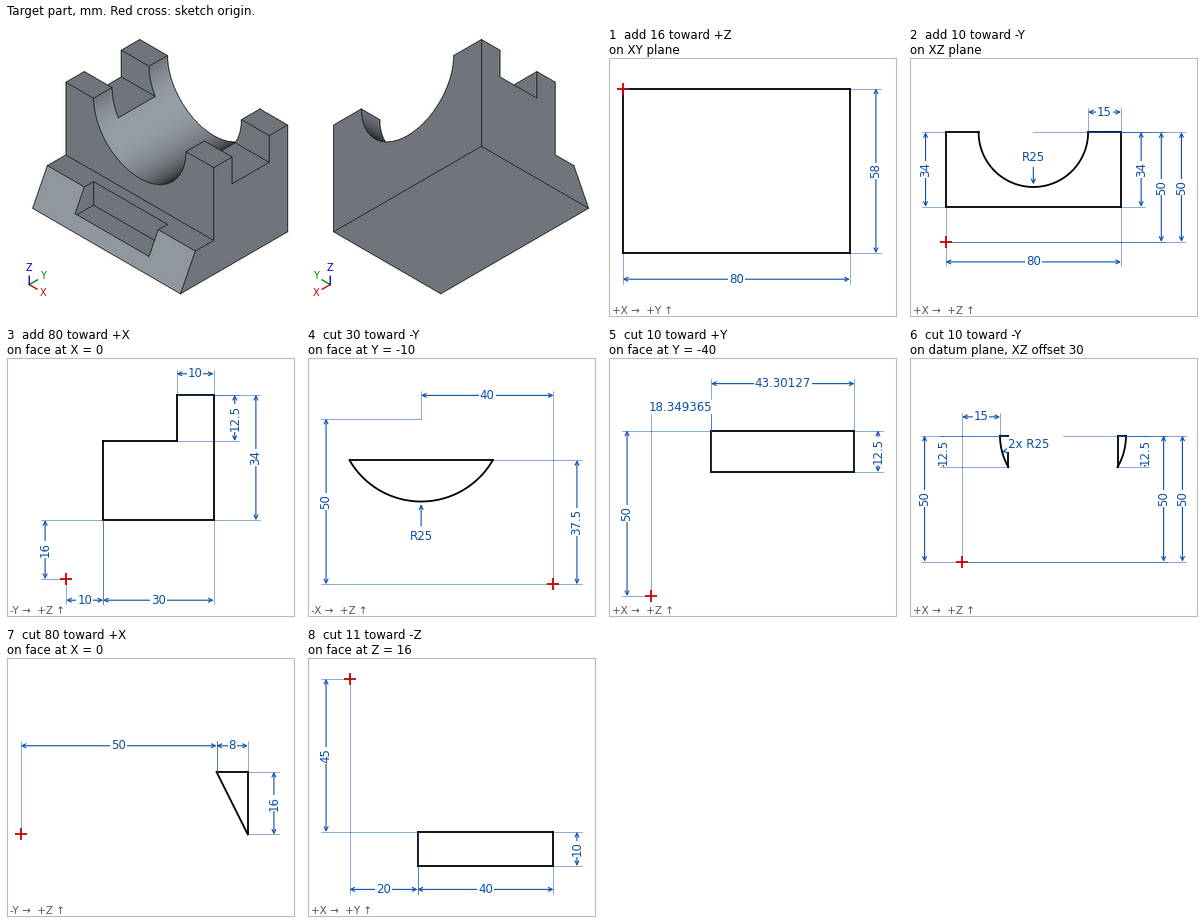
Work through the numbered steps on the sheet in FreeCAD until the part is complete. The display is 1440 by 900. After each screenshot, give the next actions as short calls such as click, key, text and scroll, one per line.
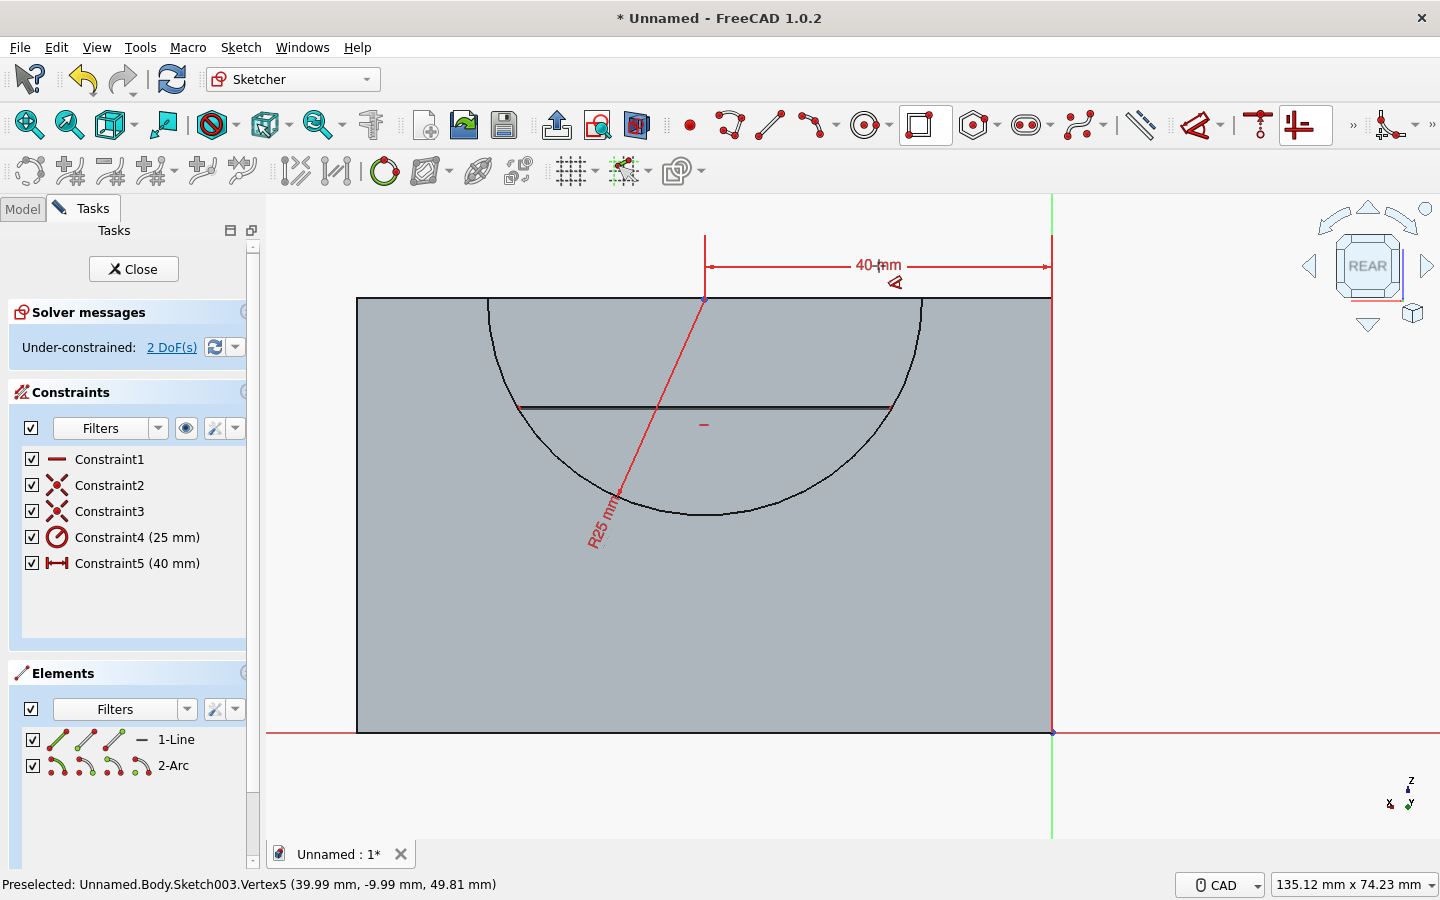
click(705, 300)
click(1086, 516)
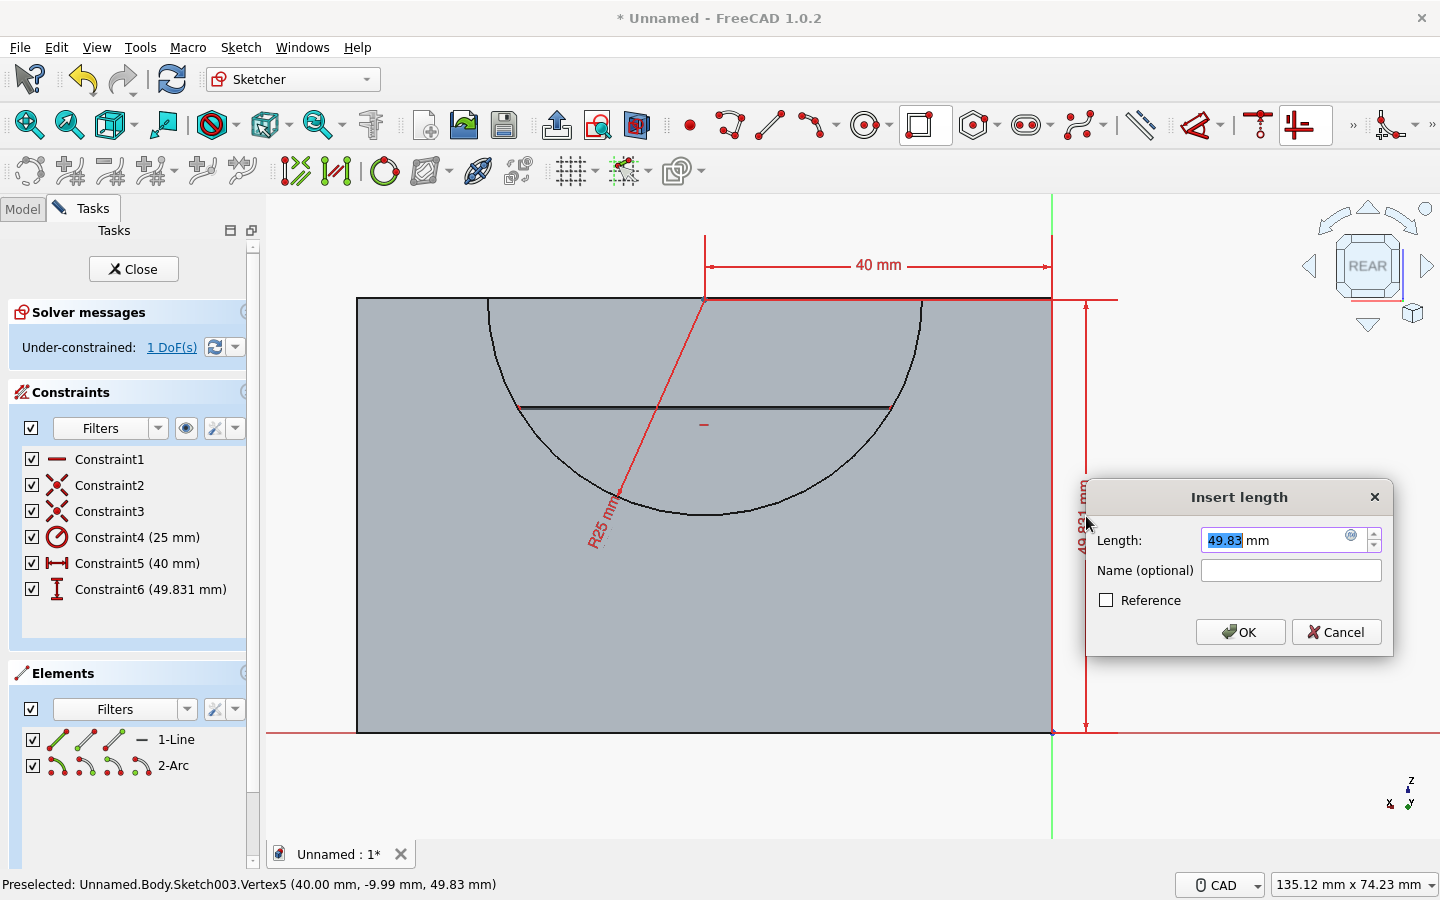
text(50)
key(Return)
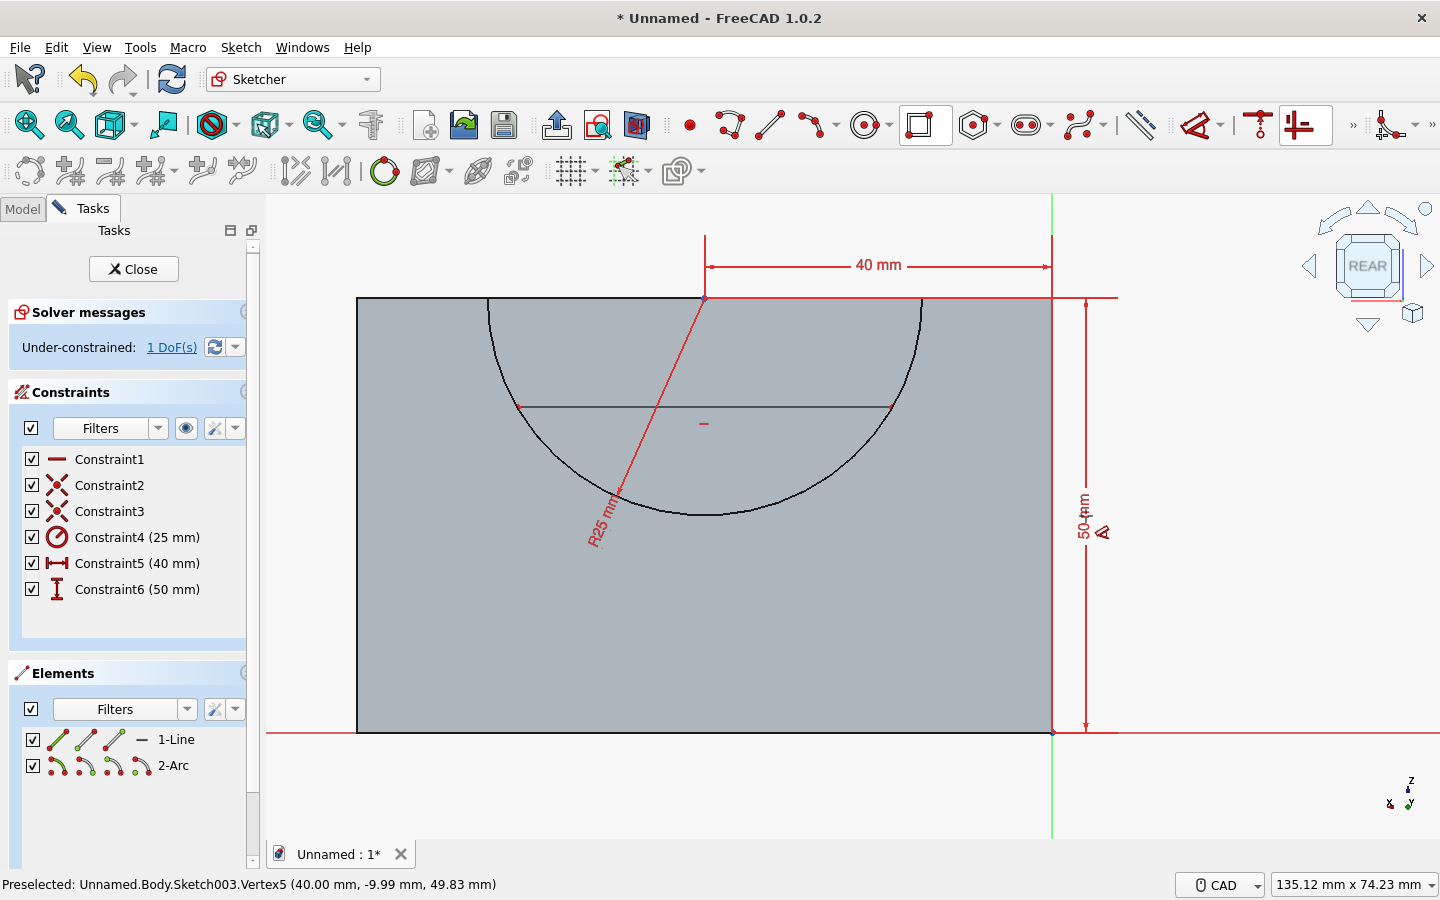
click(893, 407)
click(1086, 570)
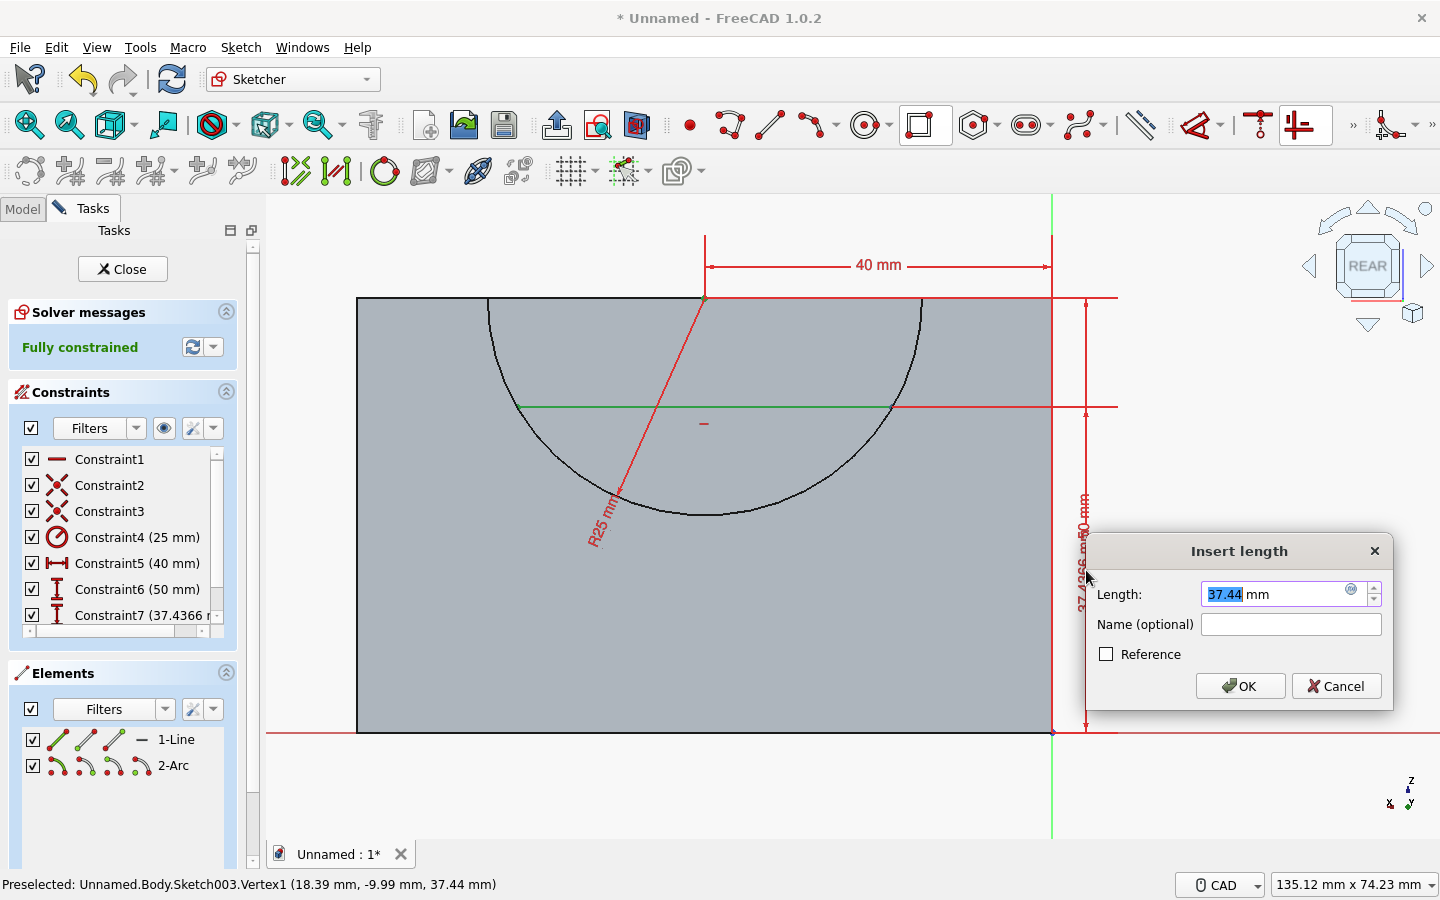
text(37.5)
key(Return)
key(Escape)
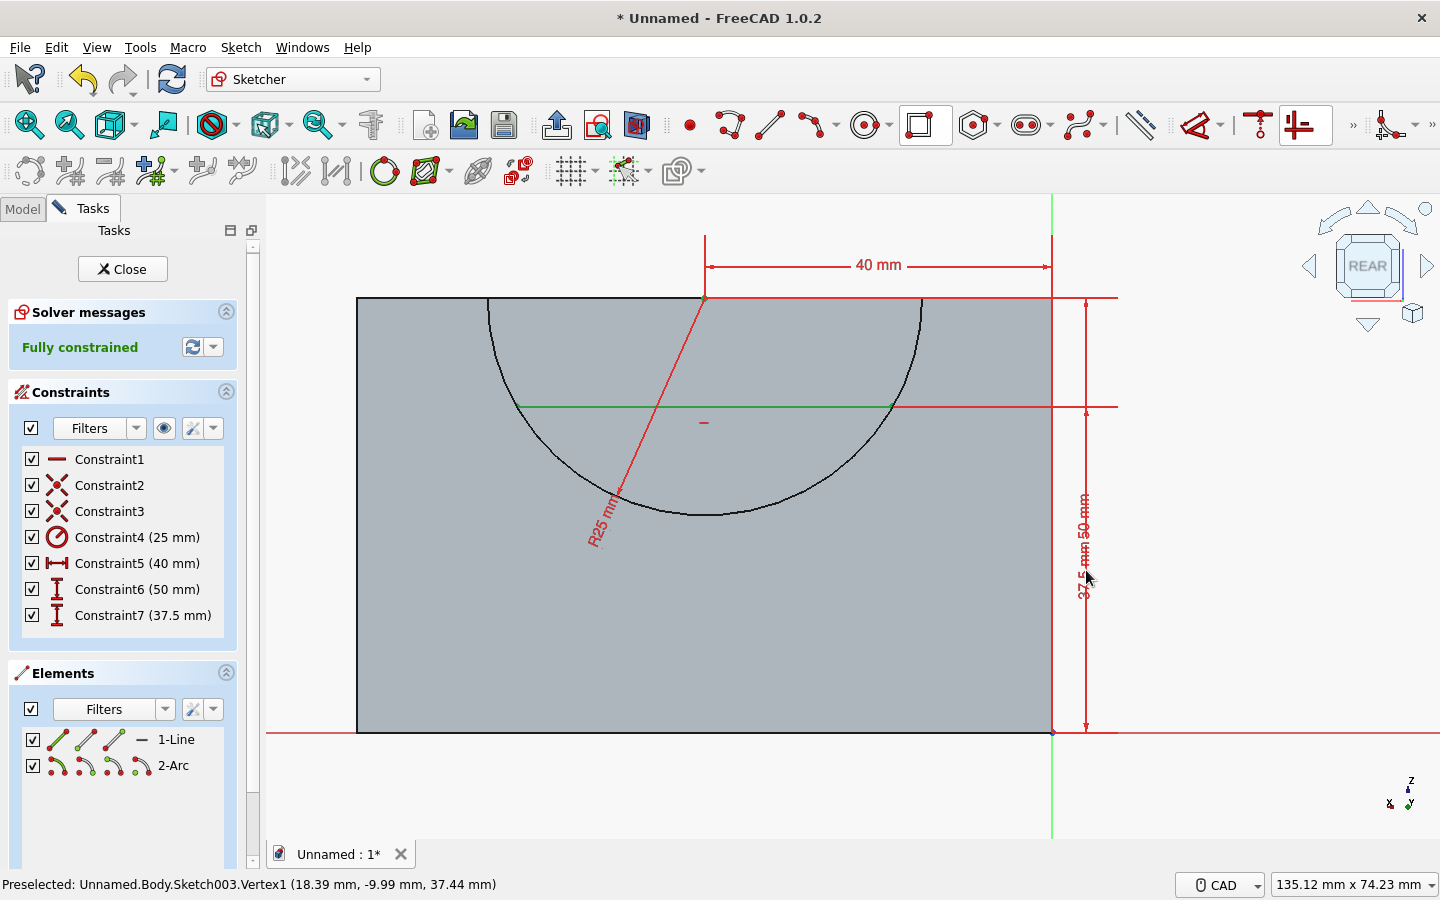
click(123, 269)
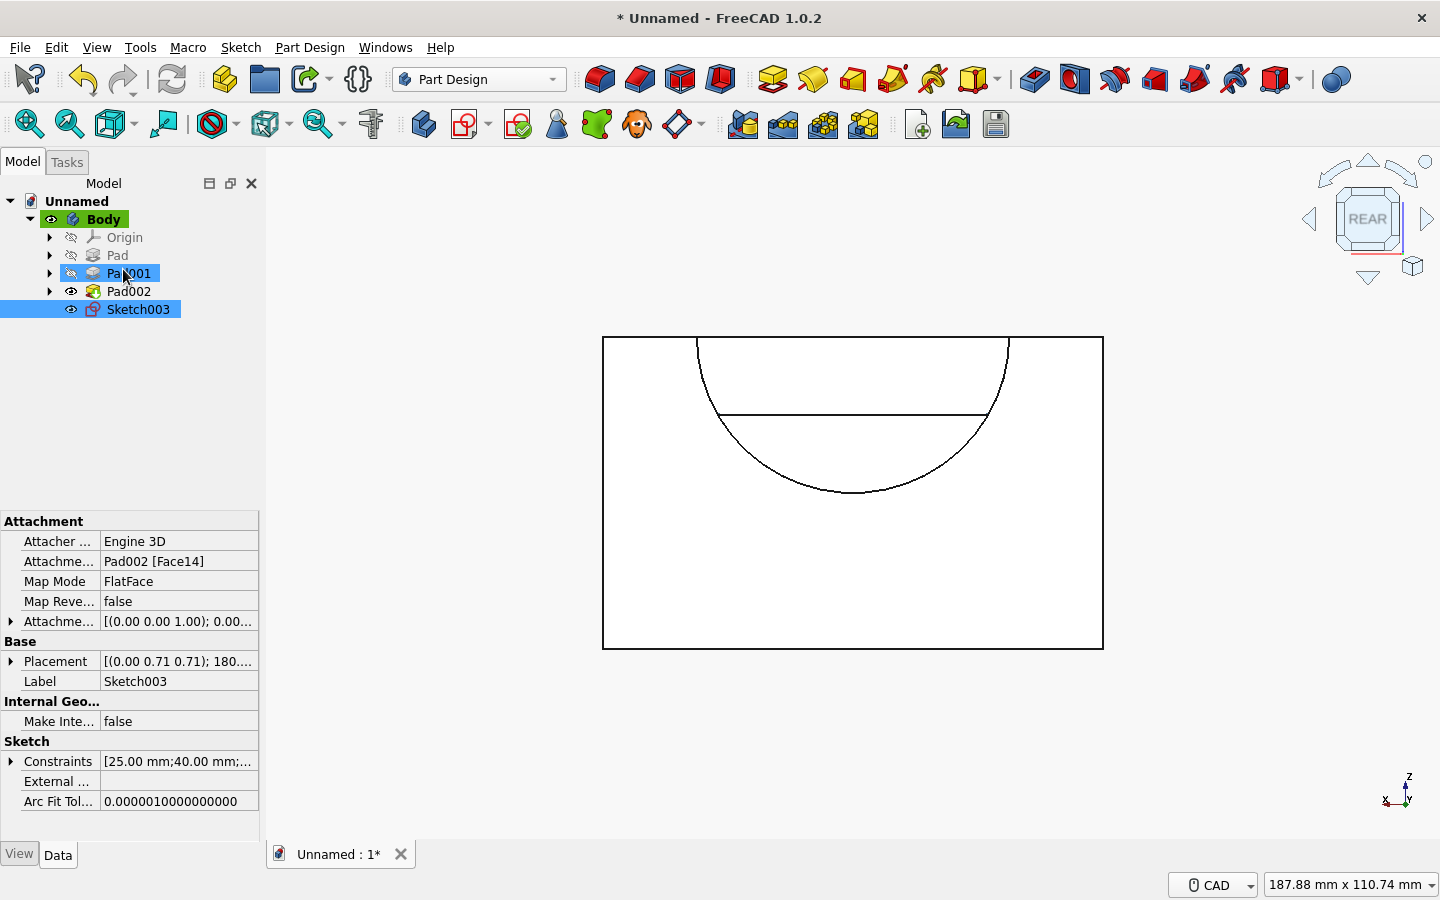
click(1036, 80)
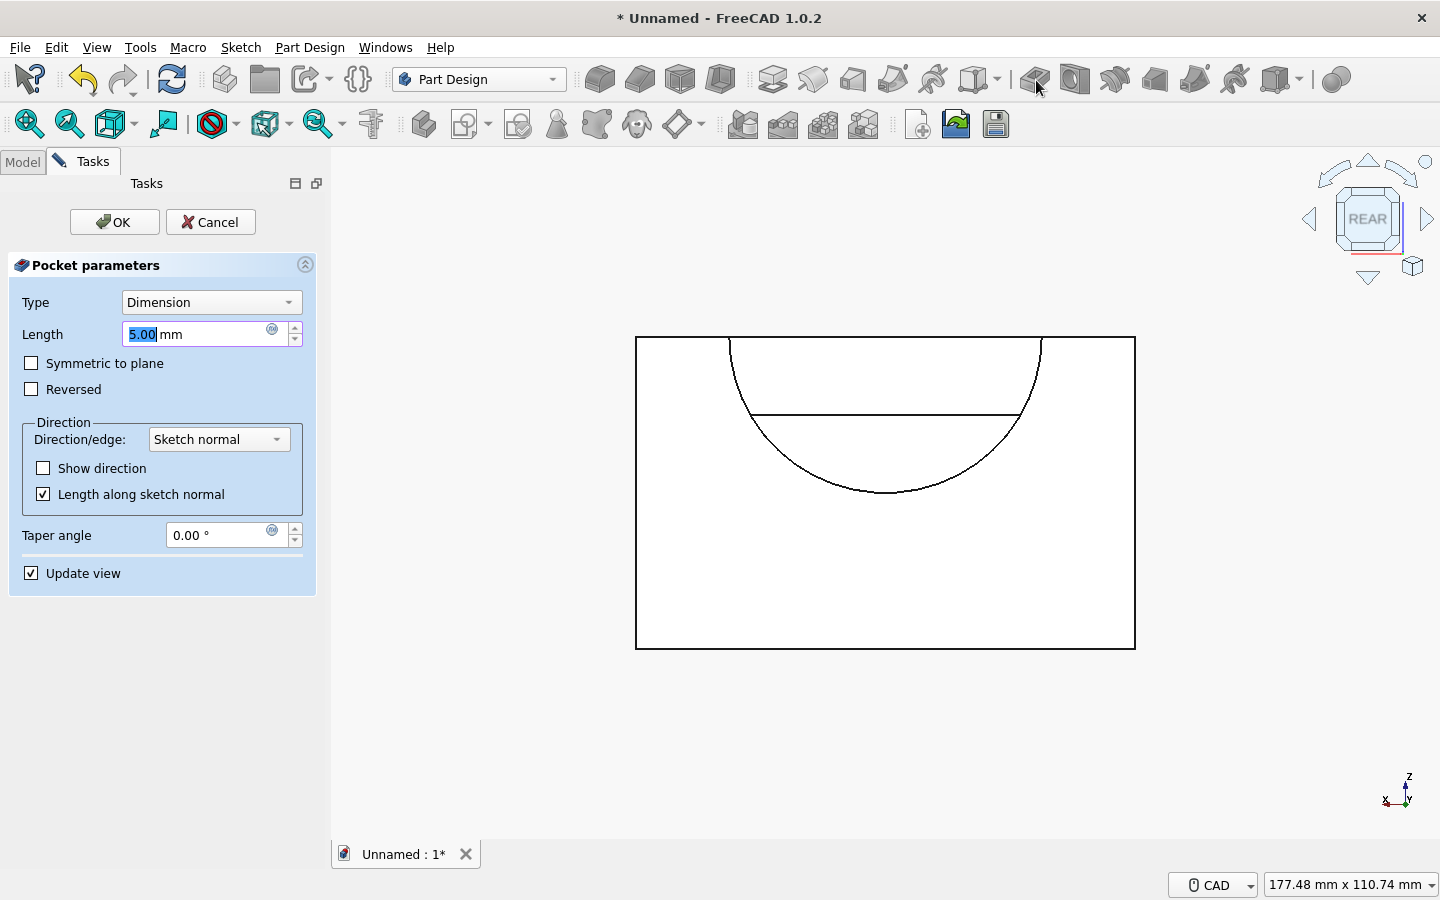
text(30)
key(Tab)